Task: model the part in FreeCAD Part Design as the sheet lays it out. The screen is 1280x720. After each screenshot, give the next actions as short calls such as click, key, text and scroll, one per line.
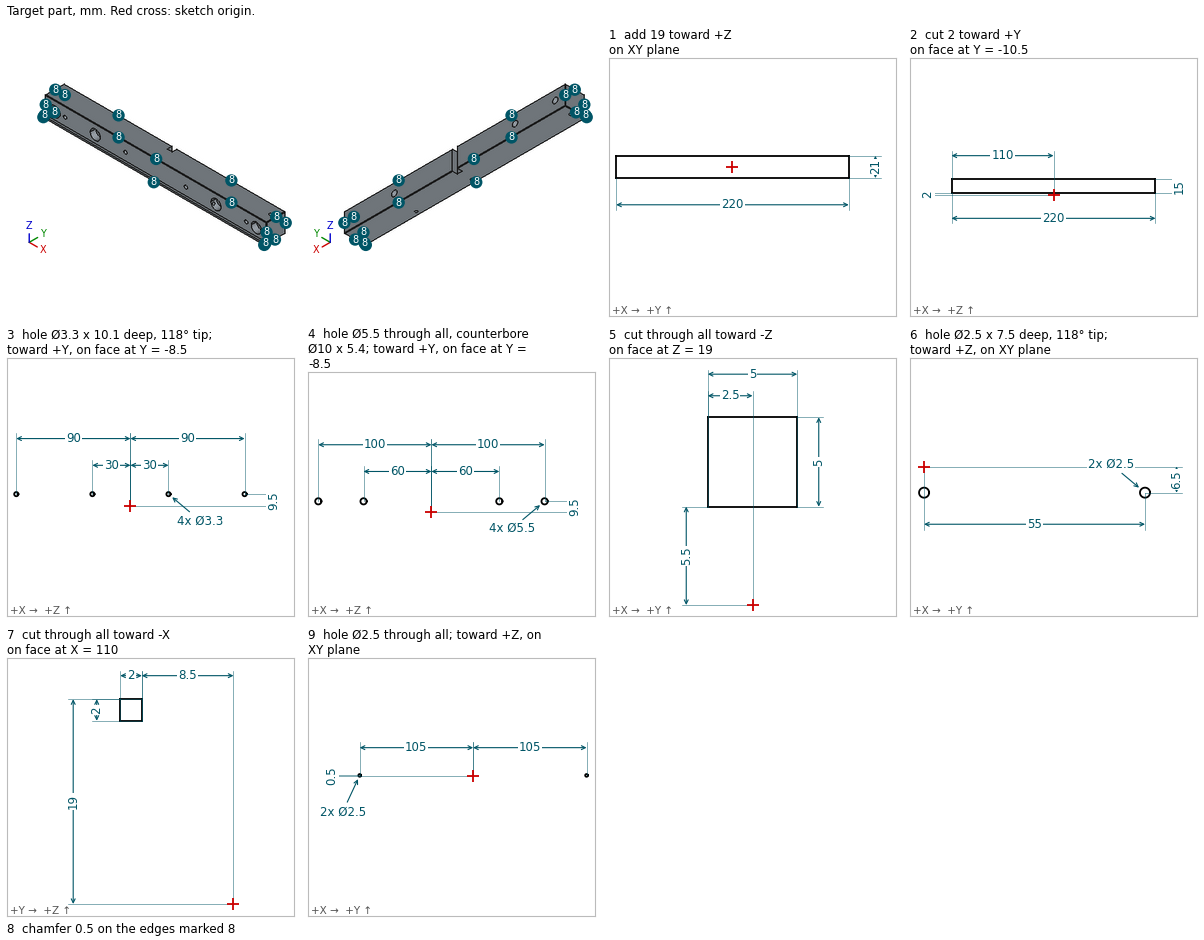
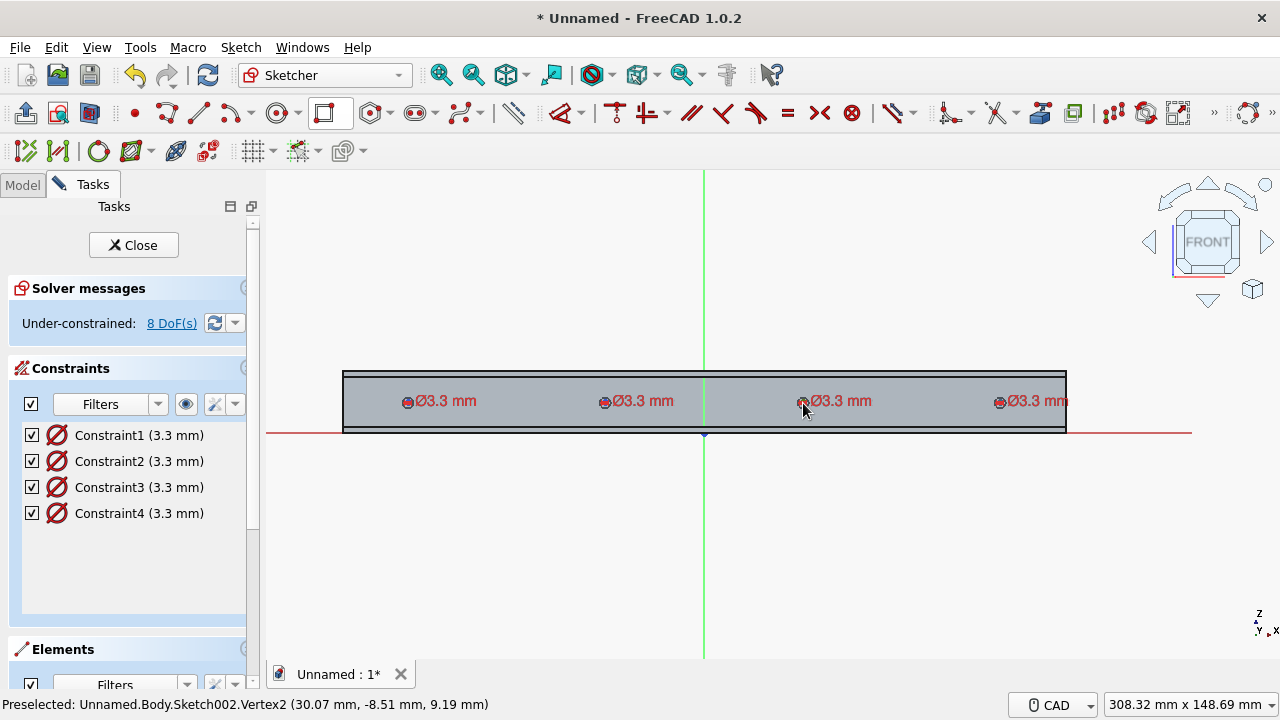
click(670, 114)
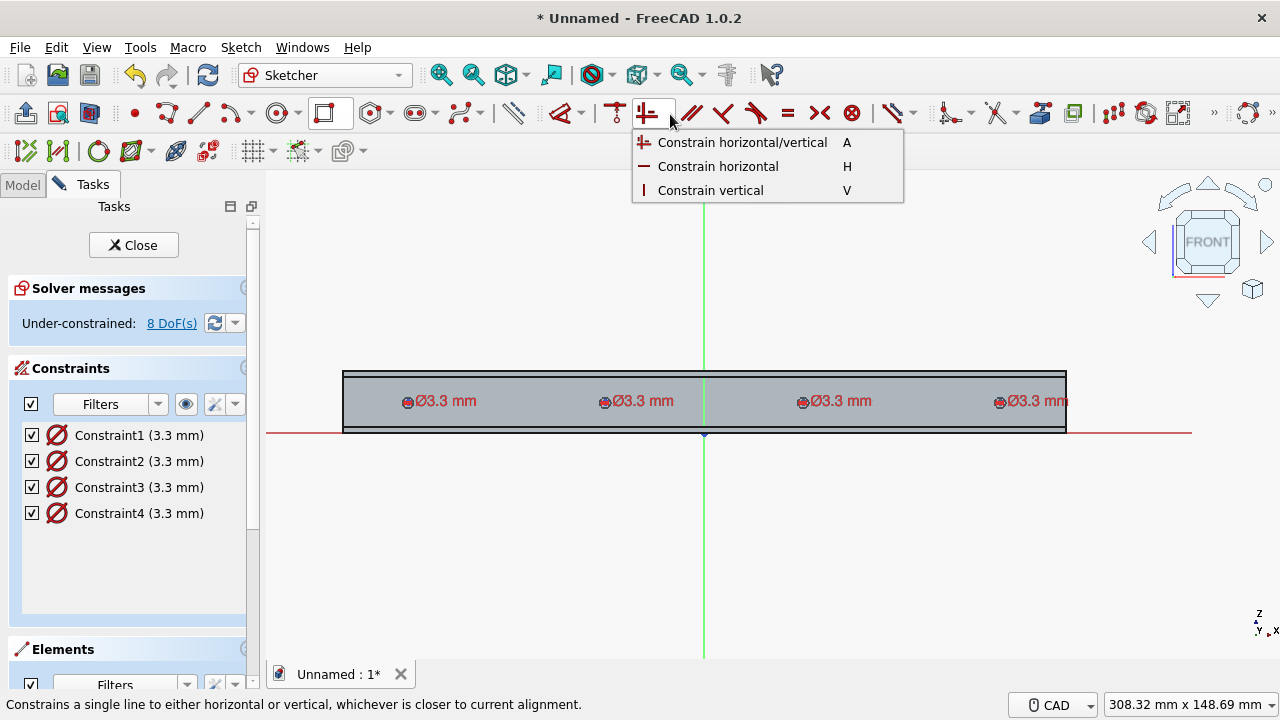
click(768, 166)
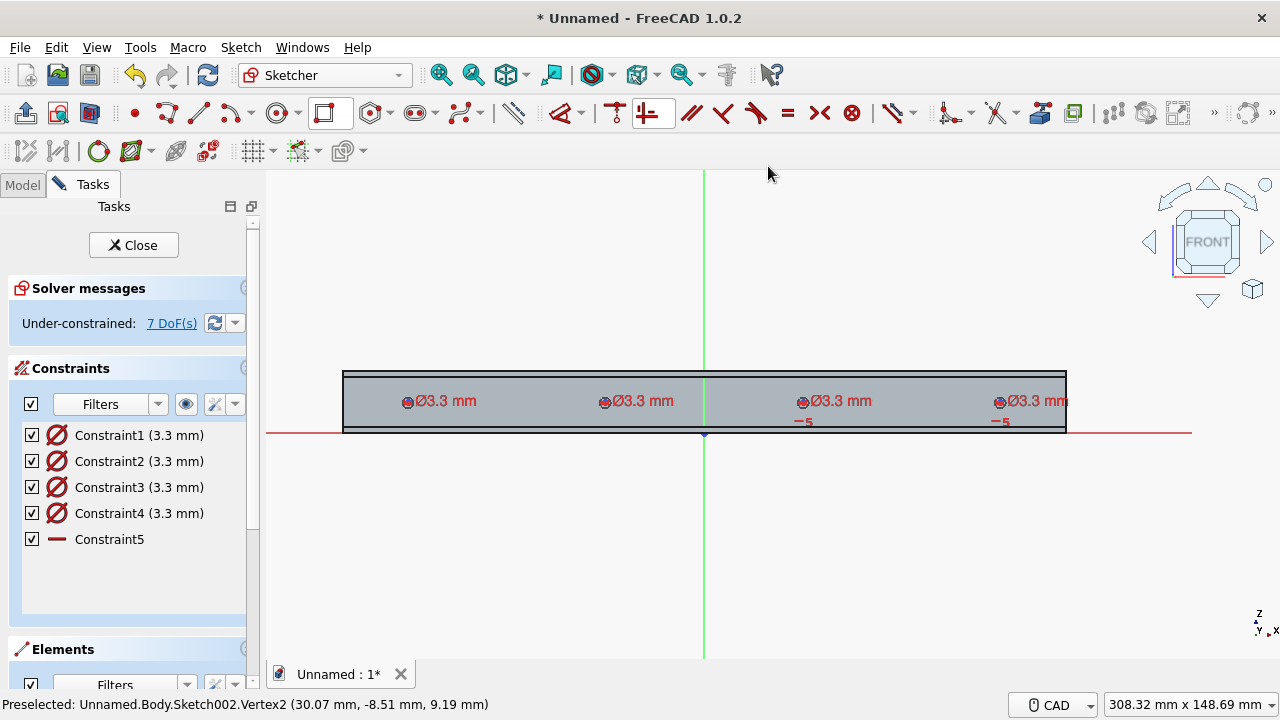
click(803, 403)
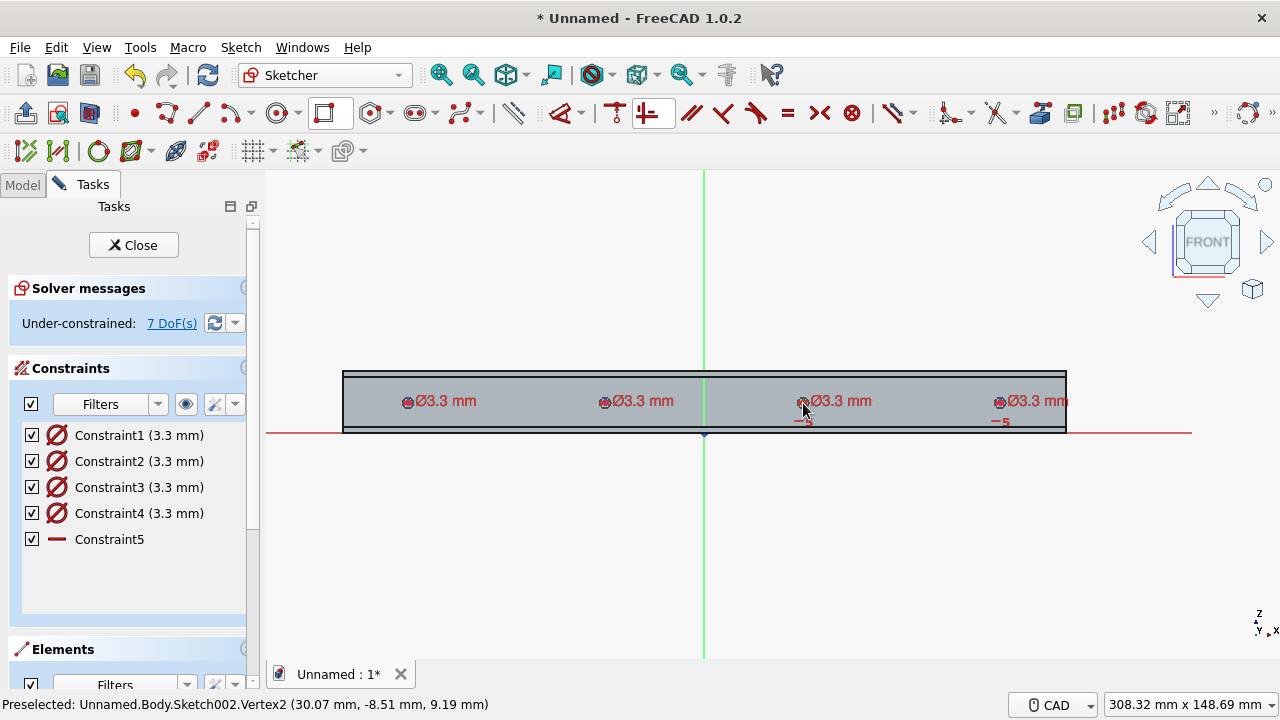
click(605, 403)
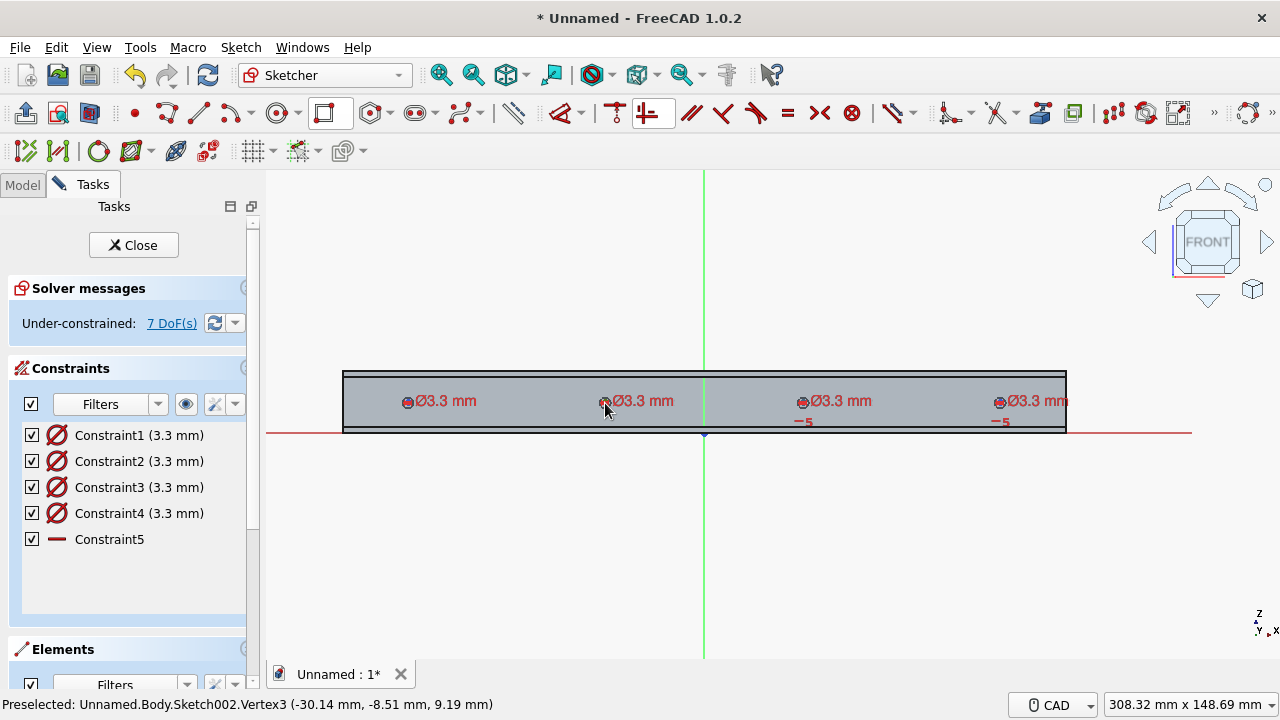
key(h)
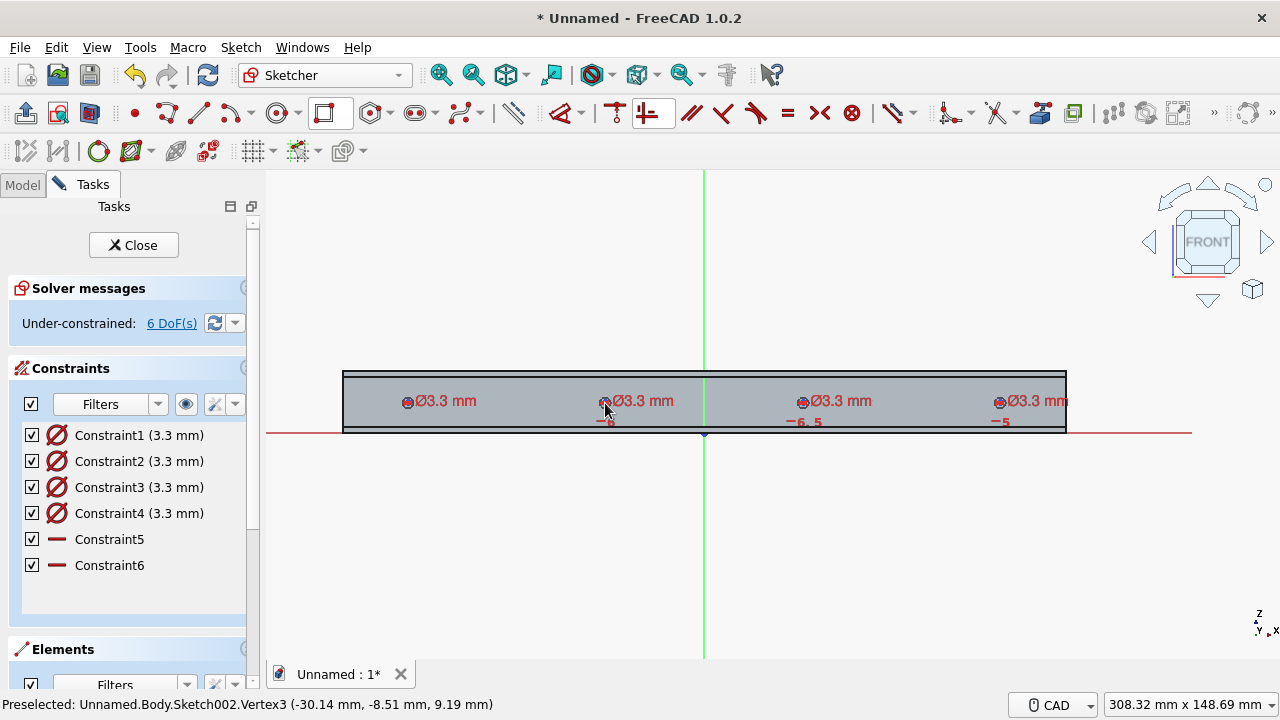
click(605, 403)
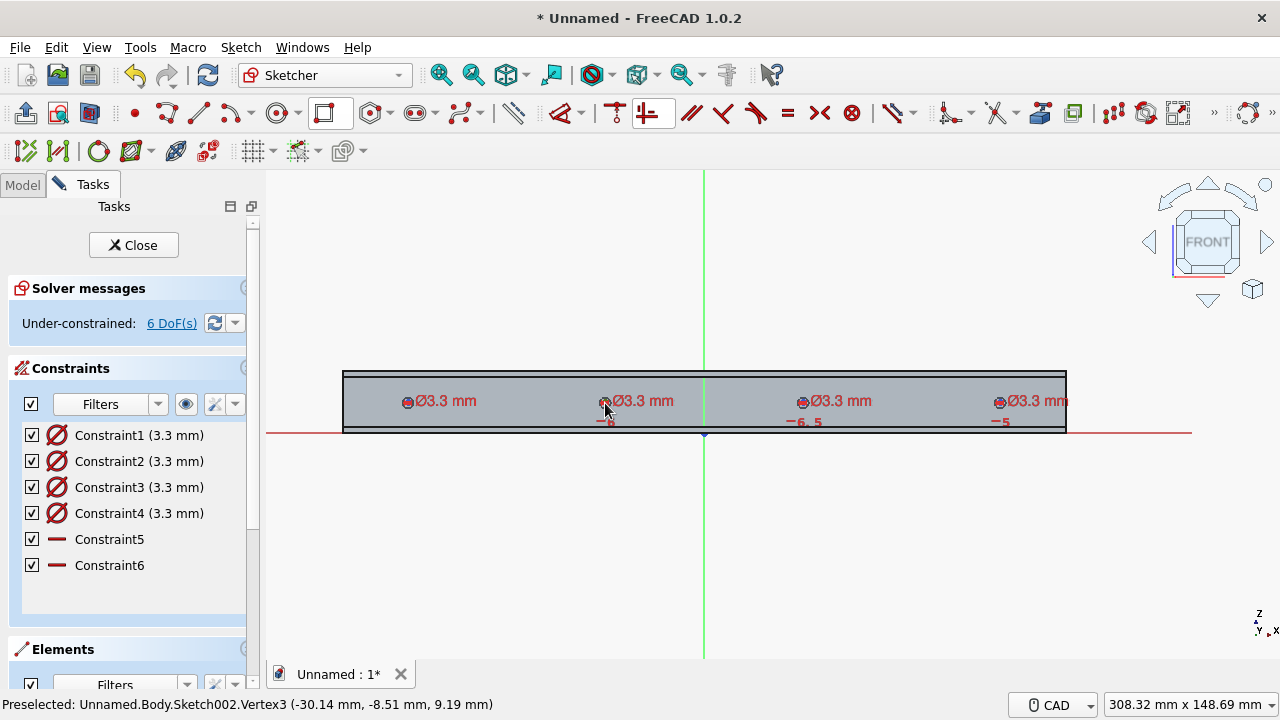
click(408, 403)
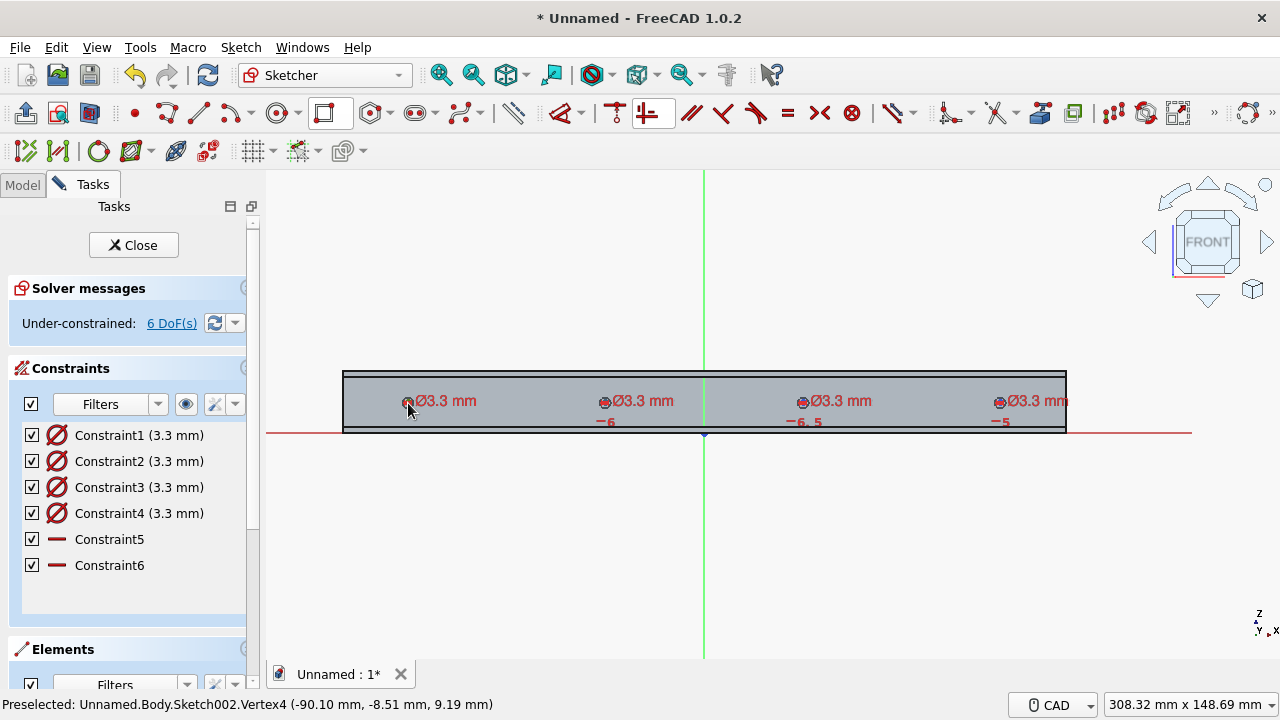
key(h)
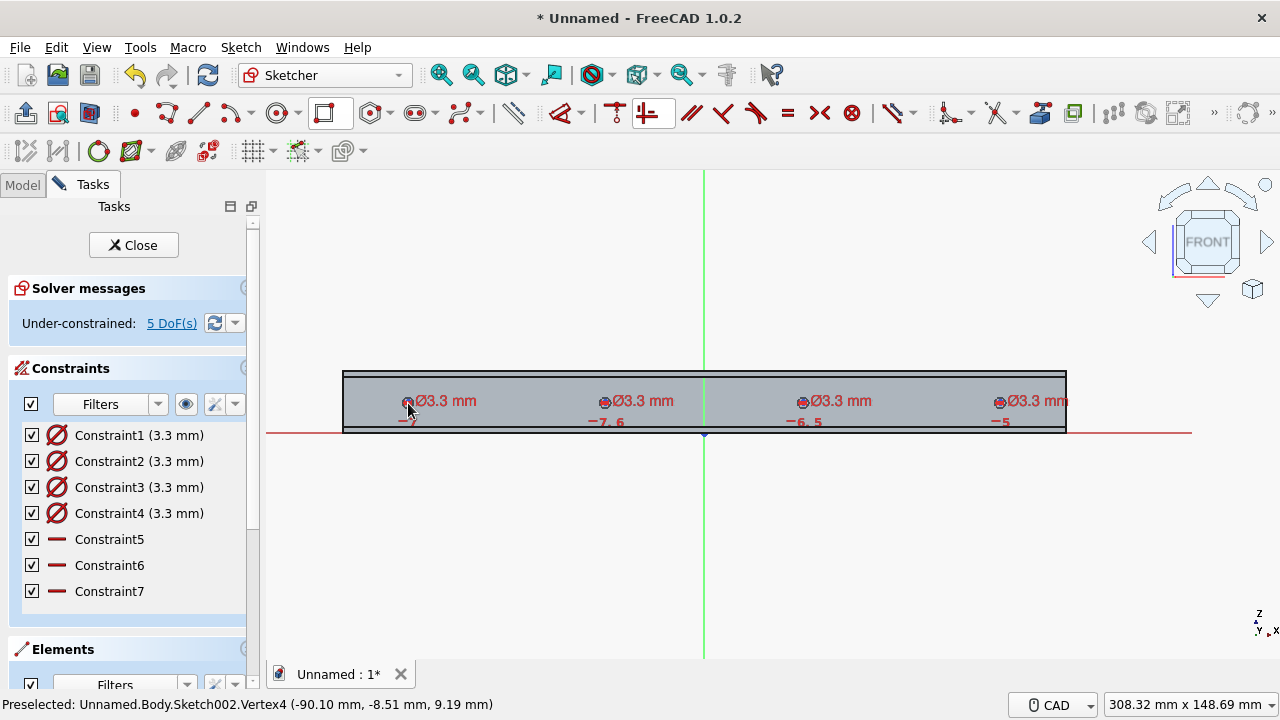
click(560, 114)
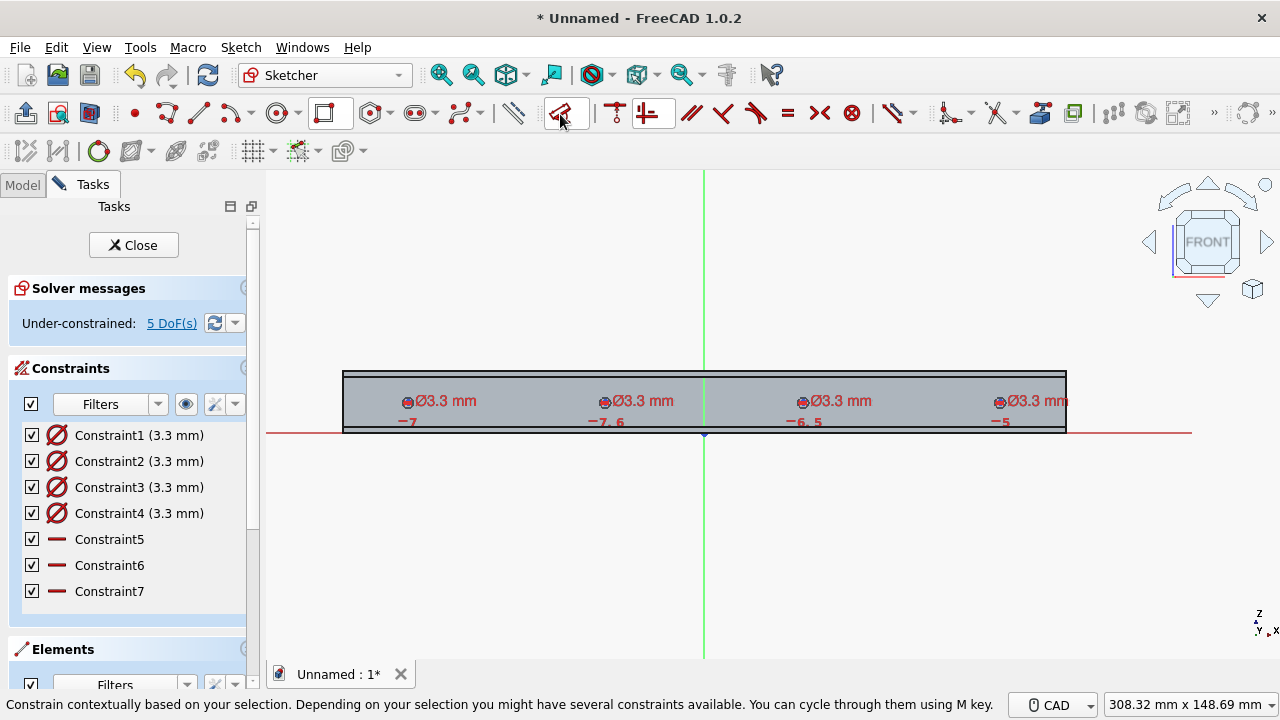
click(1000, 403)
click(852, 467)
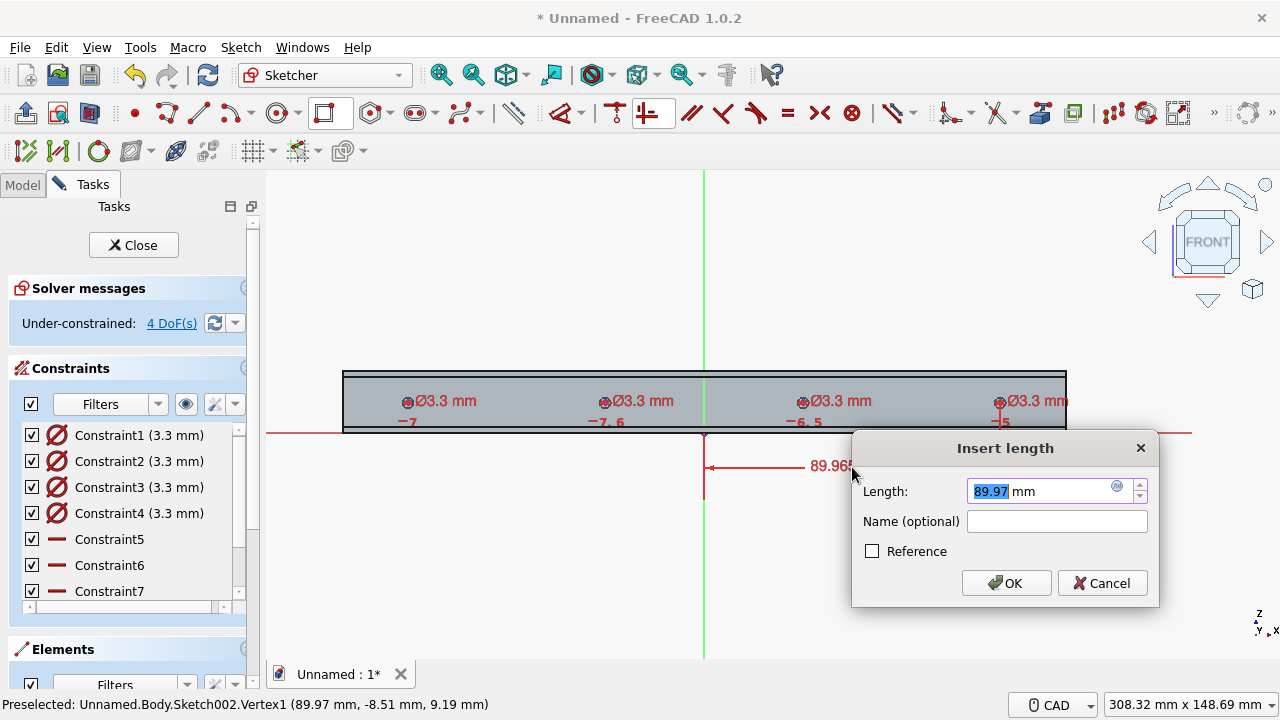
text(90)
key(Return)